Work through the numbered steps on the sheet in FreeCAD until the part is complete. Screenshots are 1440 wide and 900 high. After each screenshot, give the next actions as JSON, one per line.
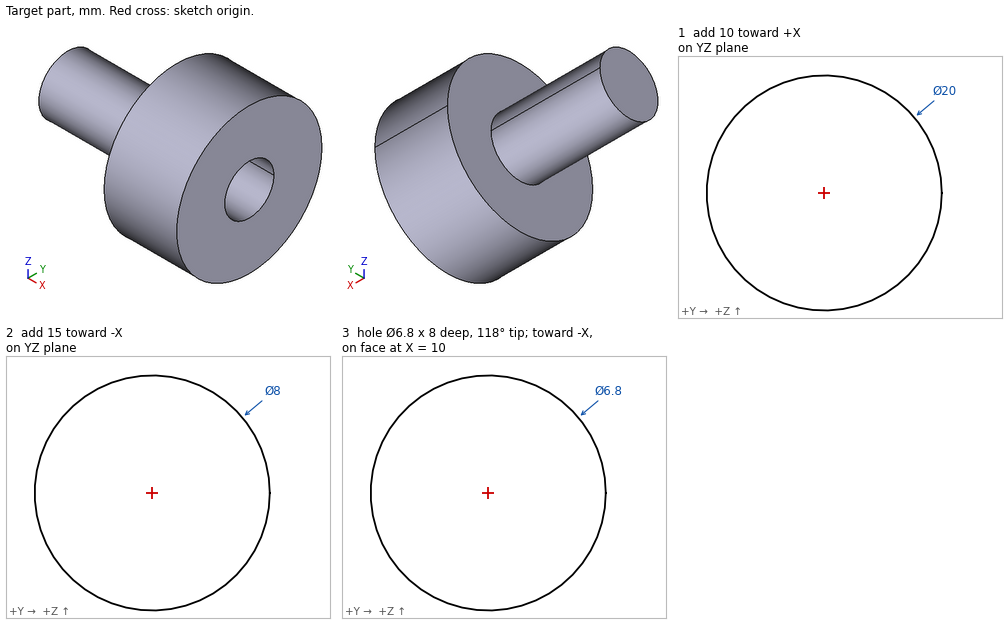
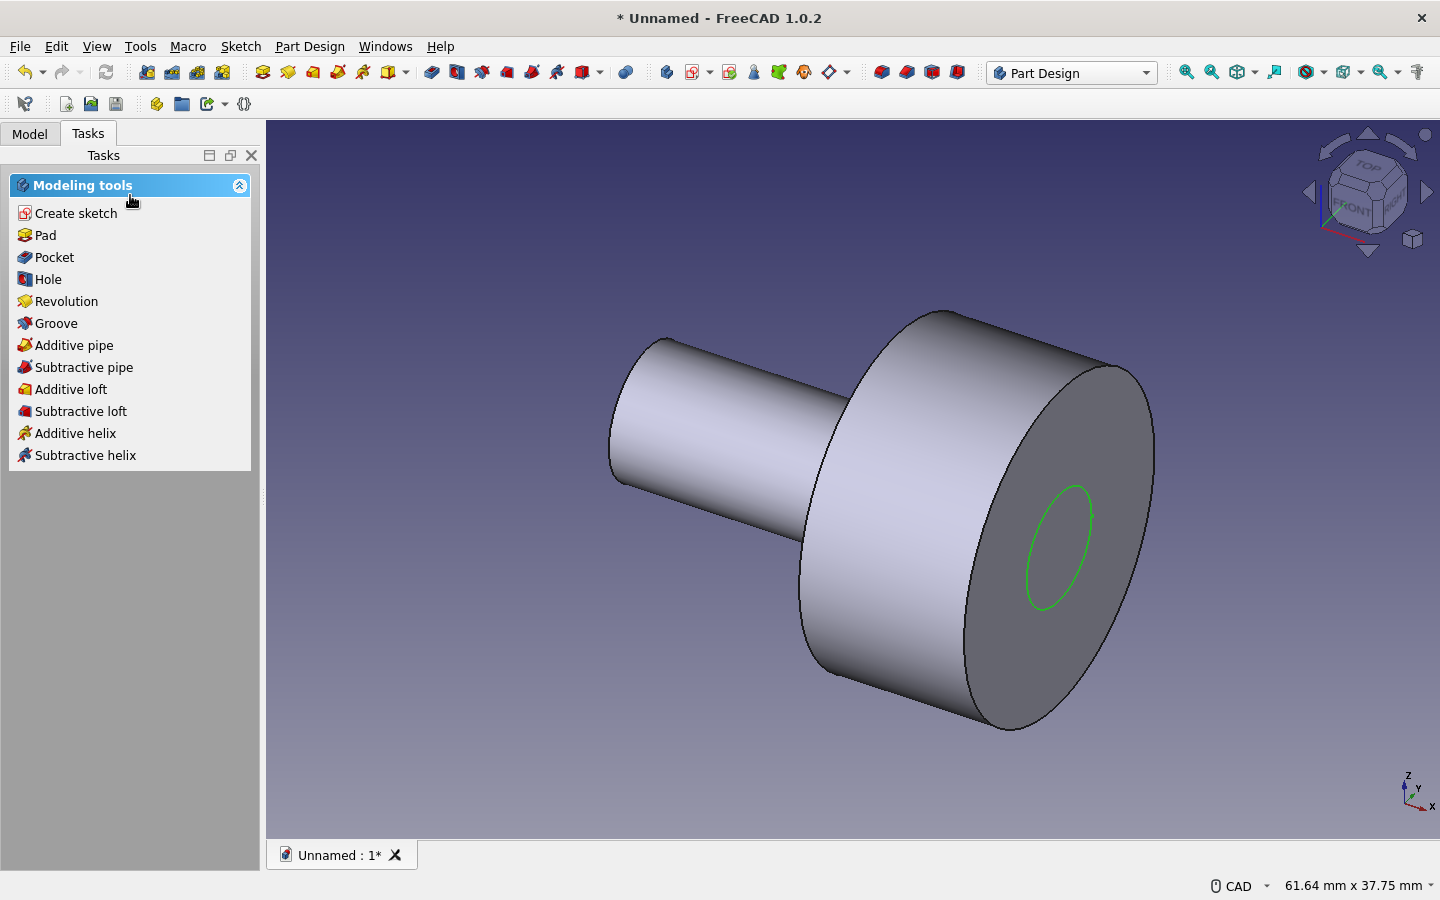
{"action": "left_click", "coordinate": [457, 72]}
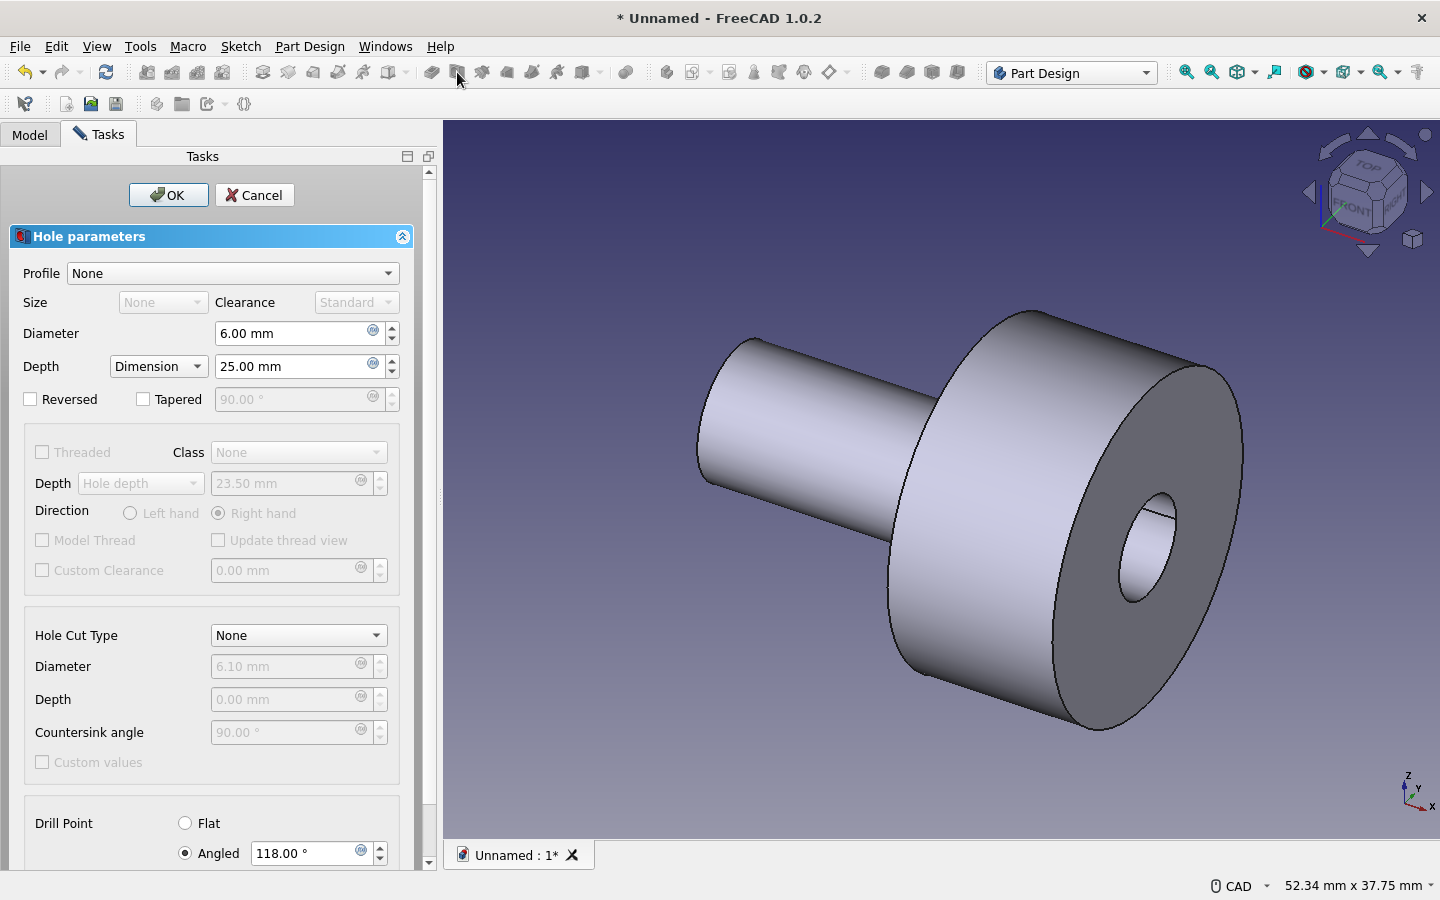
{"action": "triple_click", "coordinate": [300, 334]}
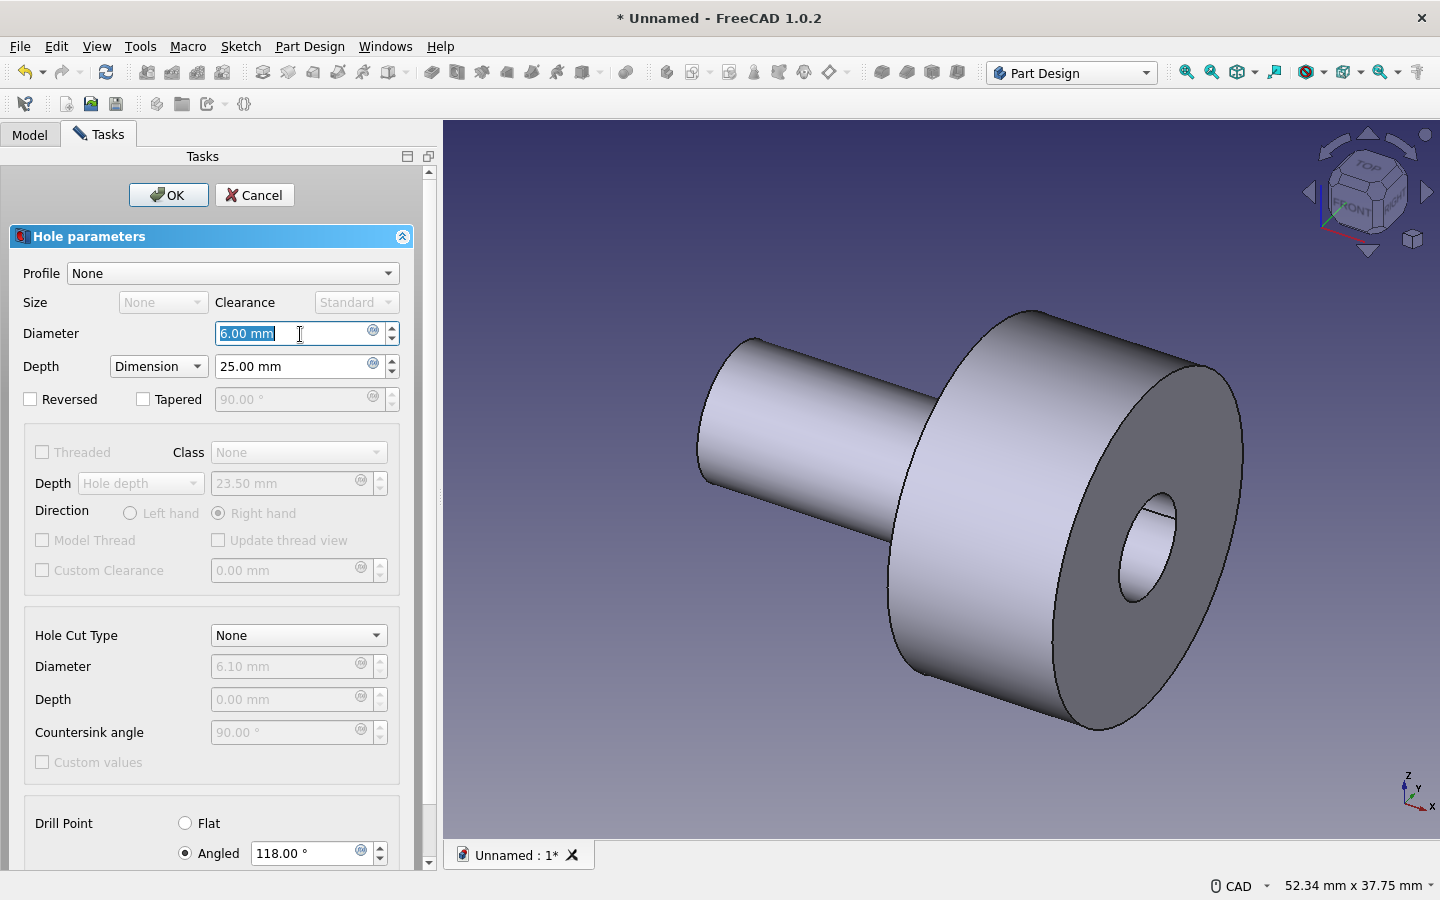
{"action": "type", "text": "6.8"}
{"action": "key", "text": "Tab"}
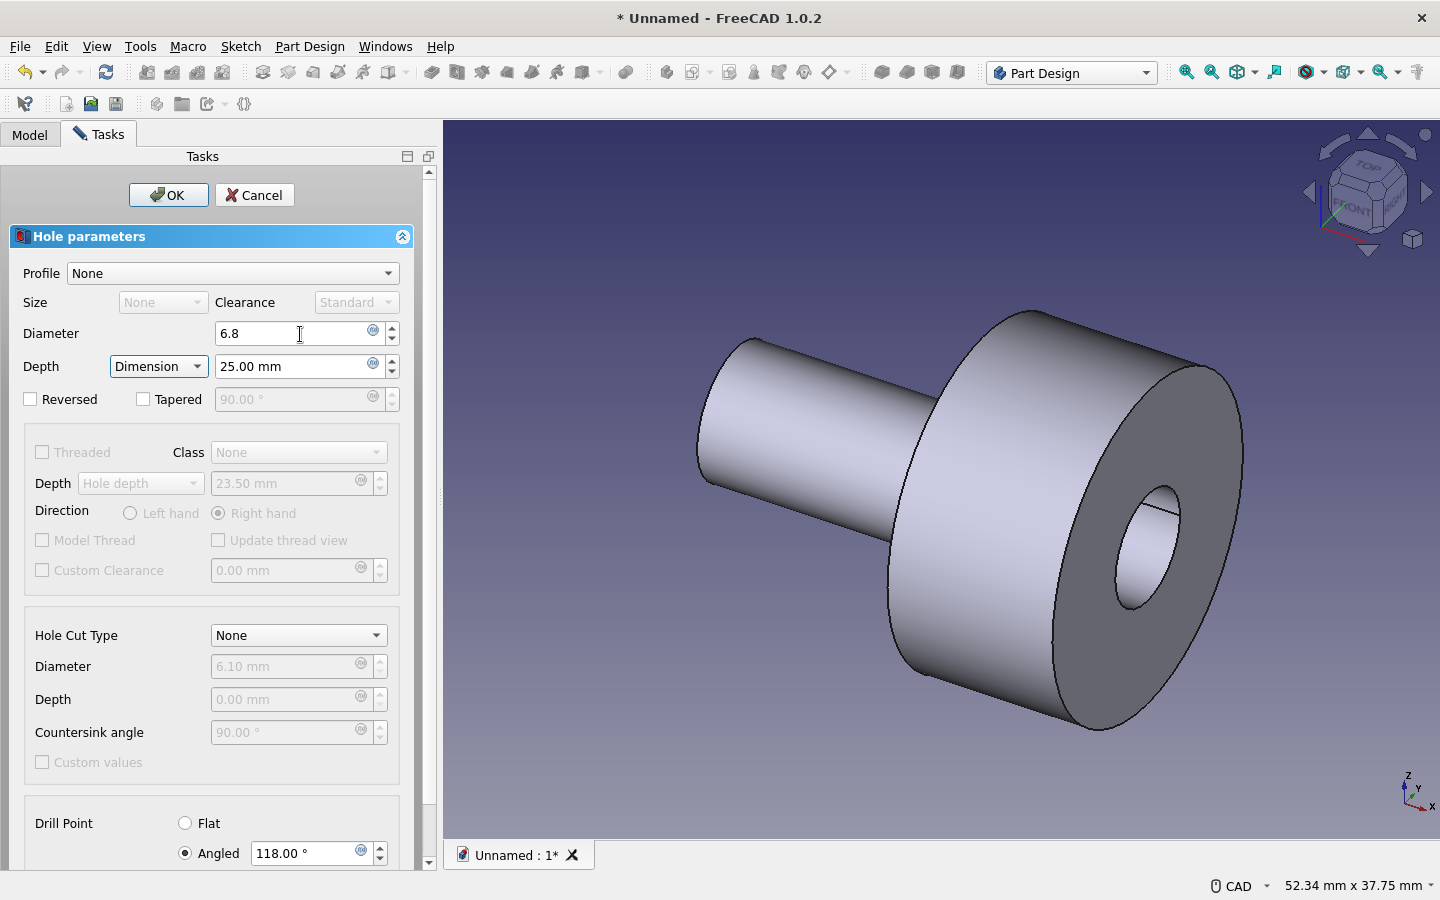
{"action": "triple_click", "coordinate": [300, 366]}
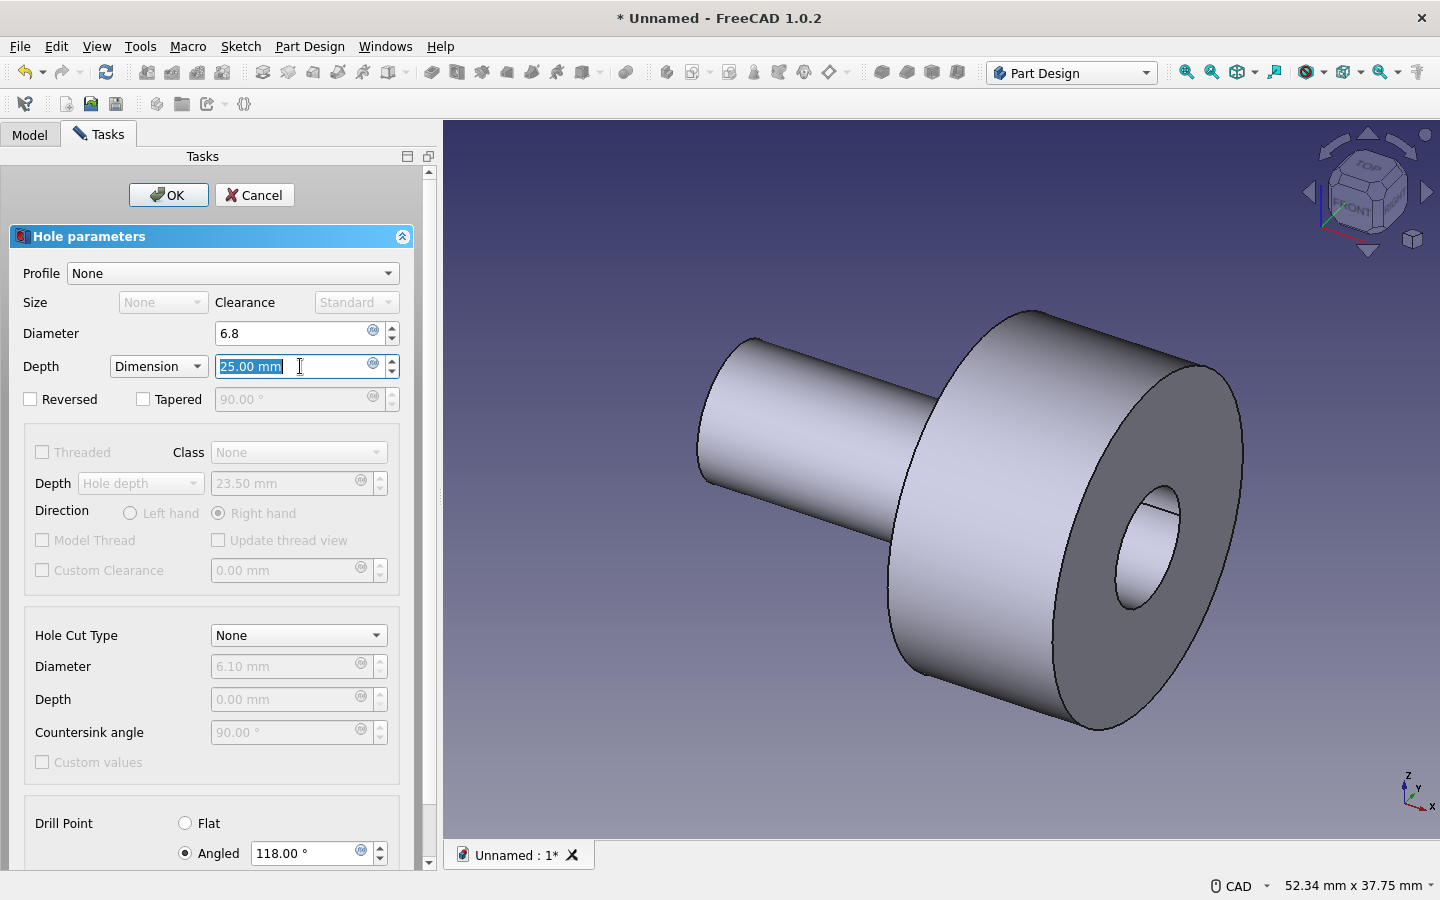
{"action": "type", "text": "8"}
{"action": "key", "text": "Tab"}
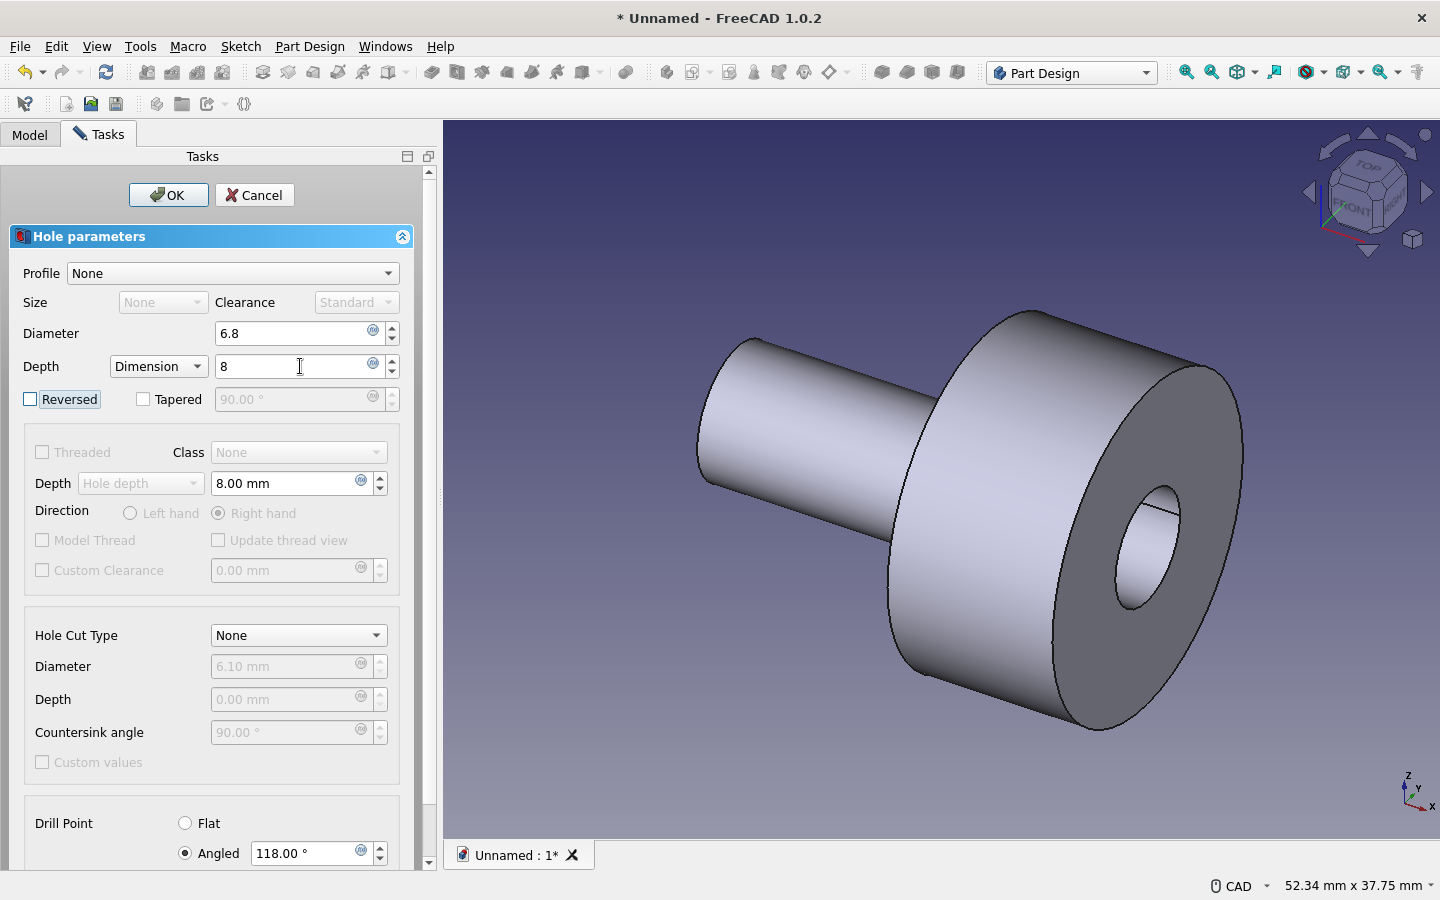
{"action": "left_click", "coordinate": [169, 195]}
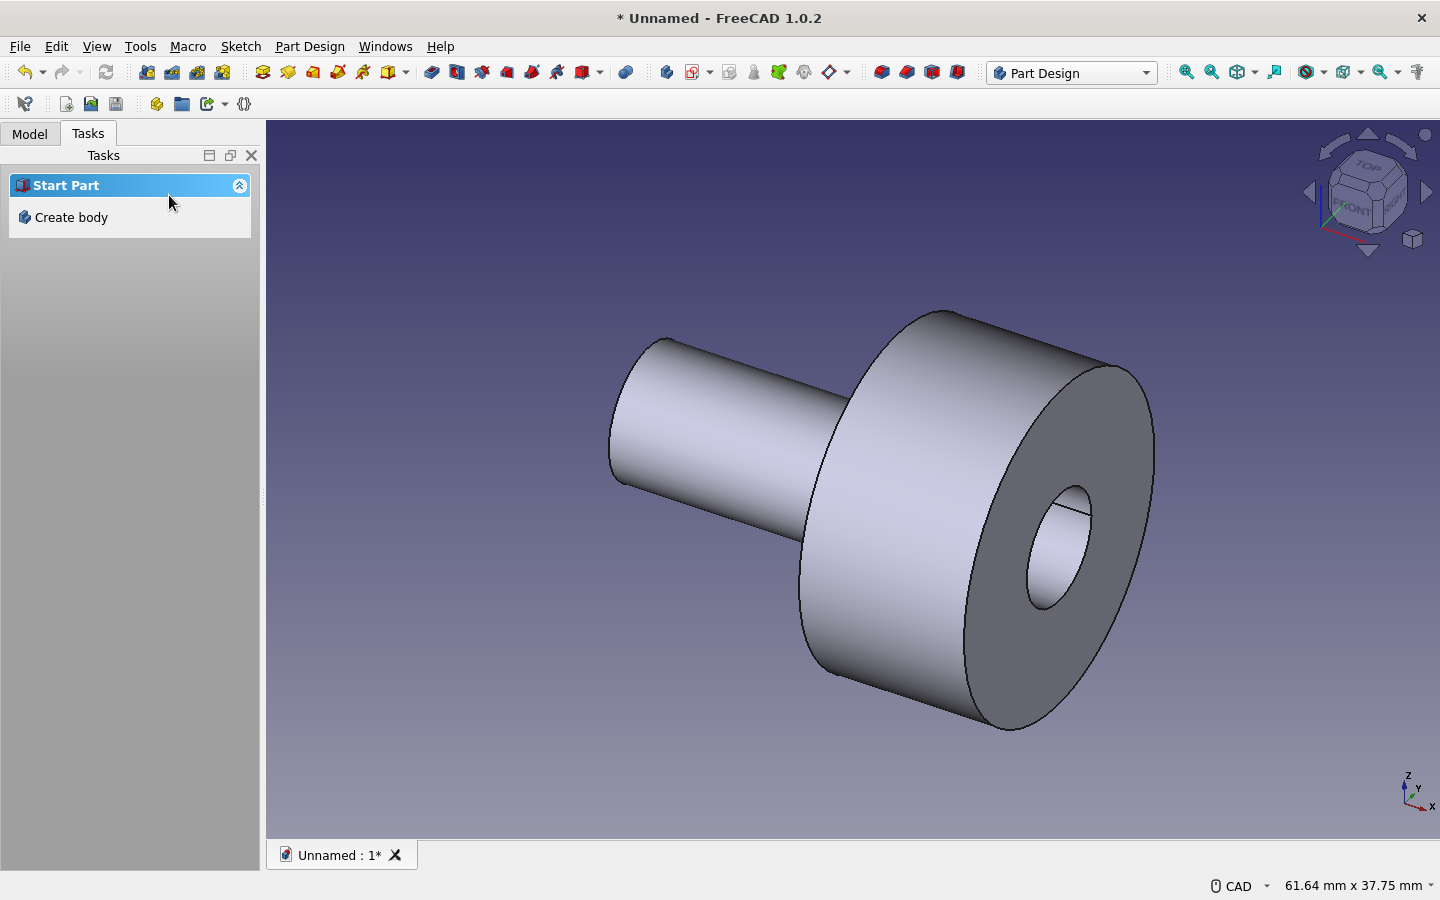
{"action": "key", "text": "0"}